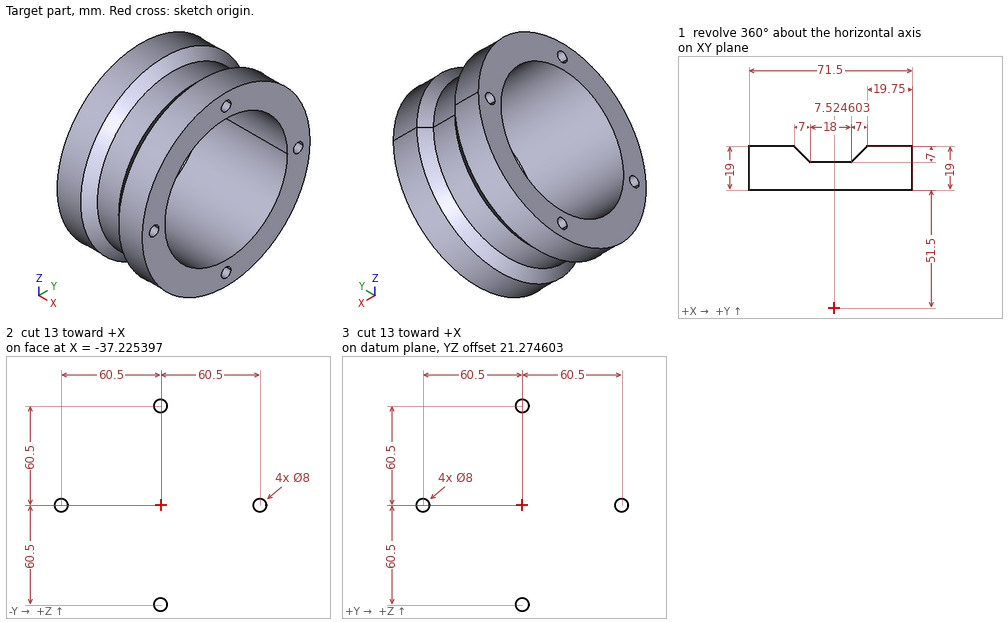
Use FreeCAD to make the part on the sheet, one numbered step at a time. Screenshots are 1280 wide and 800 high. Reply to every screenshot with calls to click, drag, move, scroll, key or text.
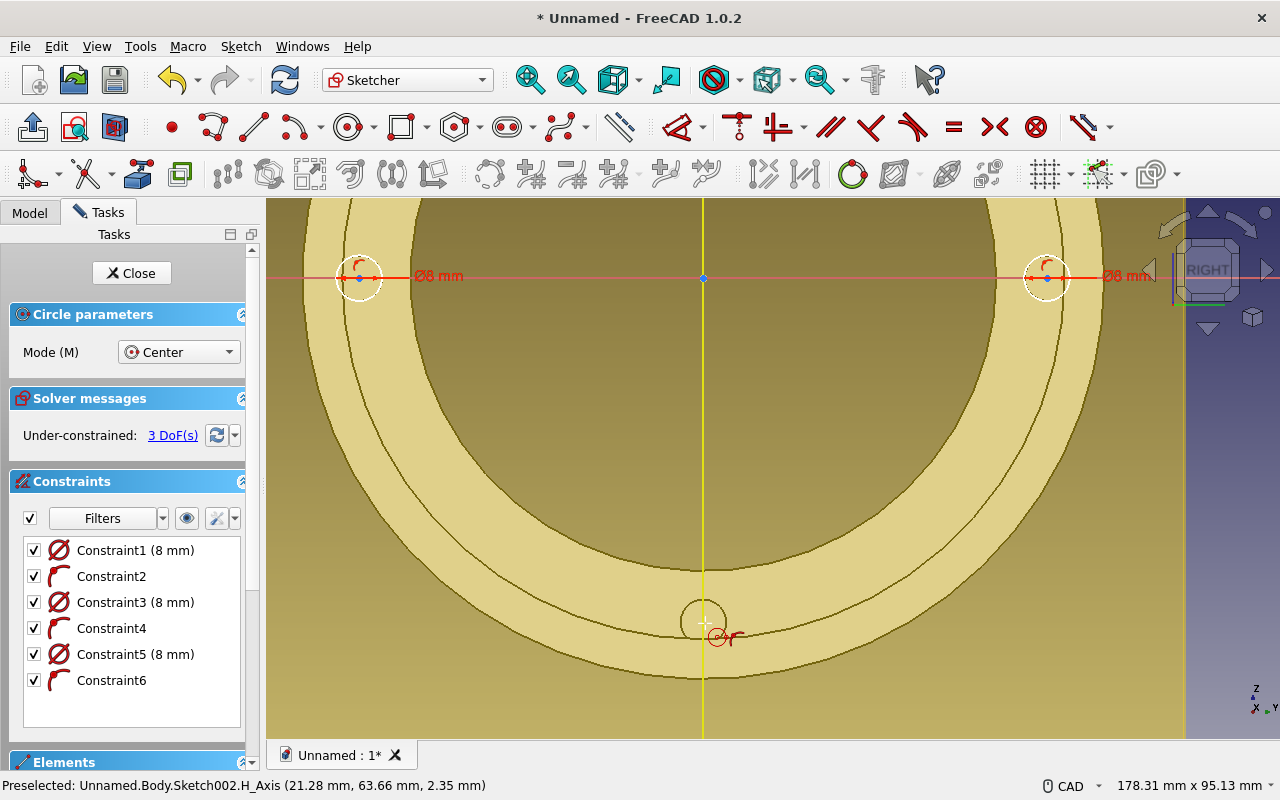
click(703, 622)
move(719, 606)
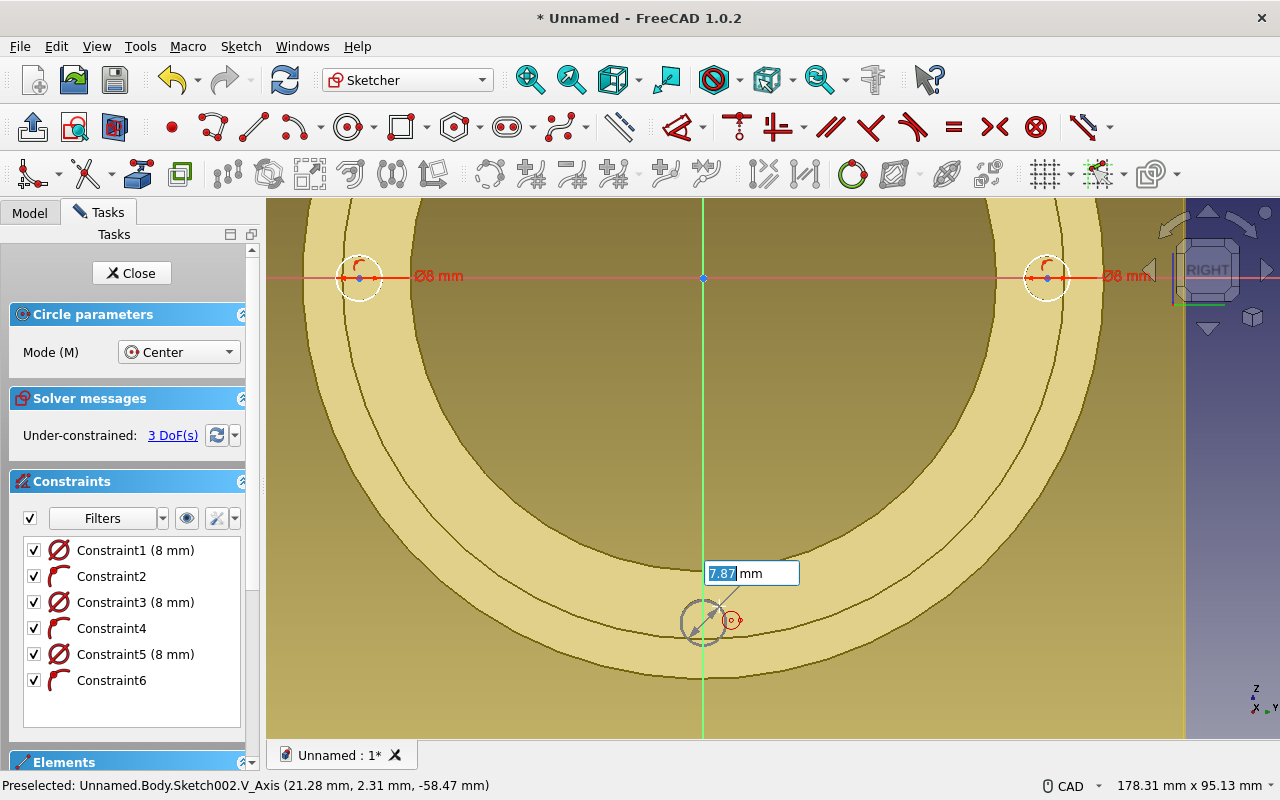
text(8)
key(Return)
key(Escape)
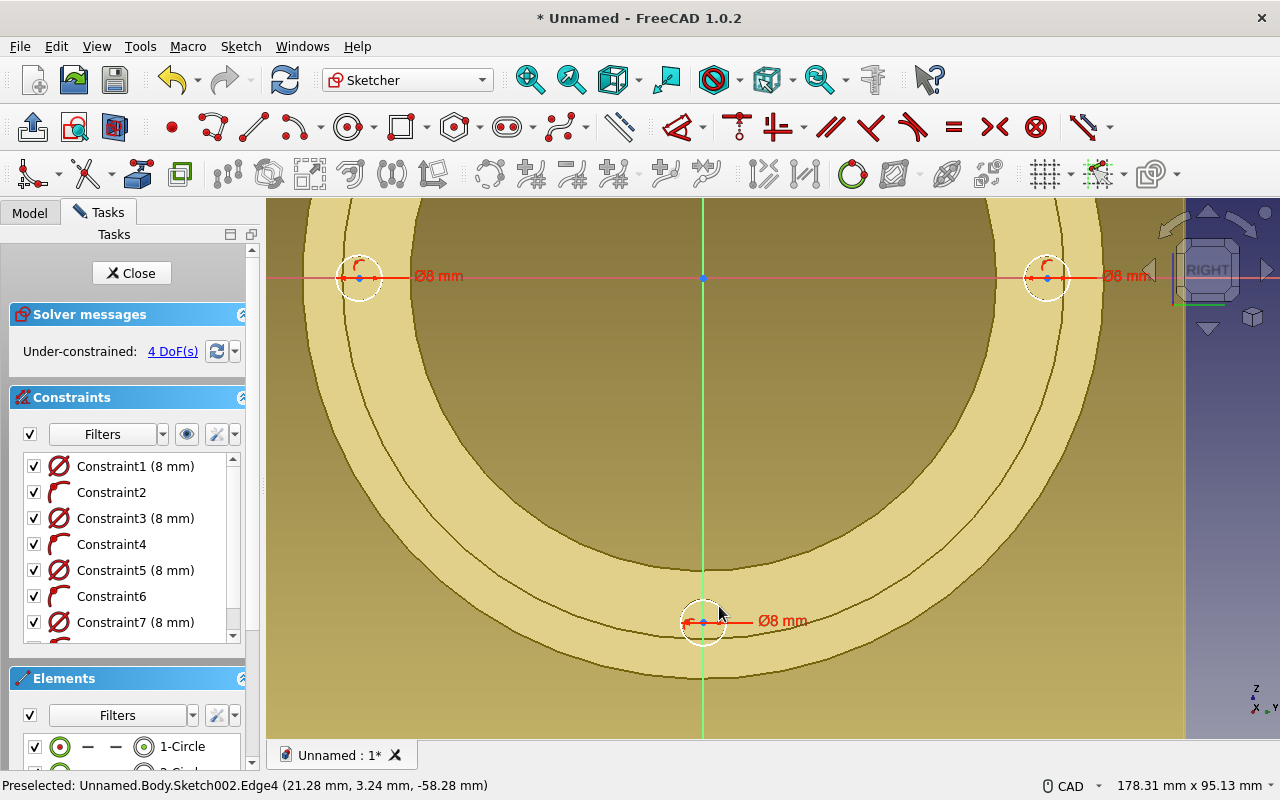
click(676, 128)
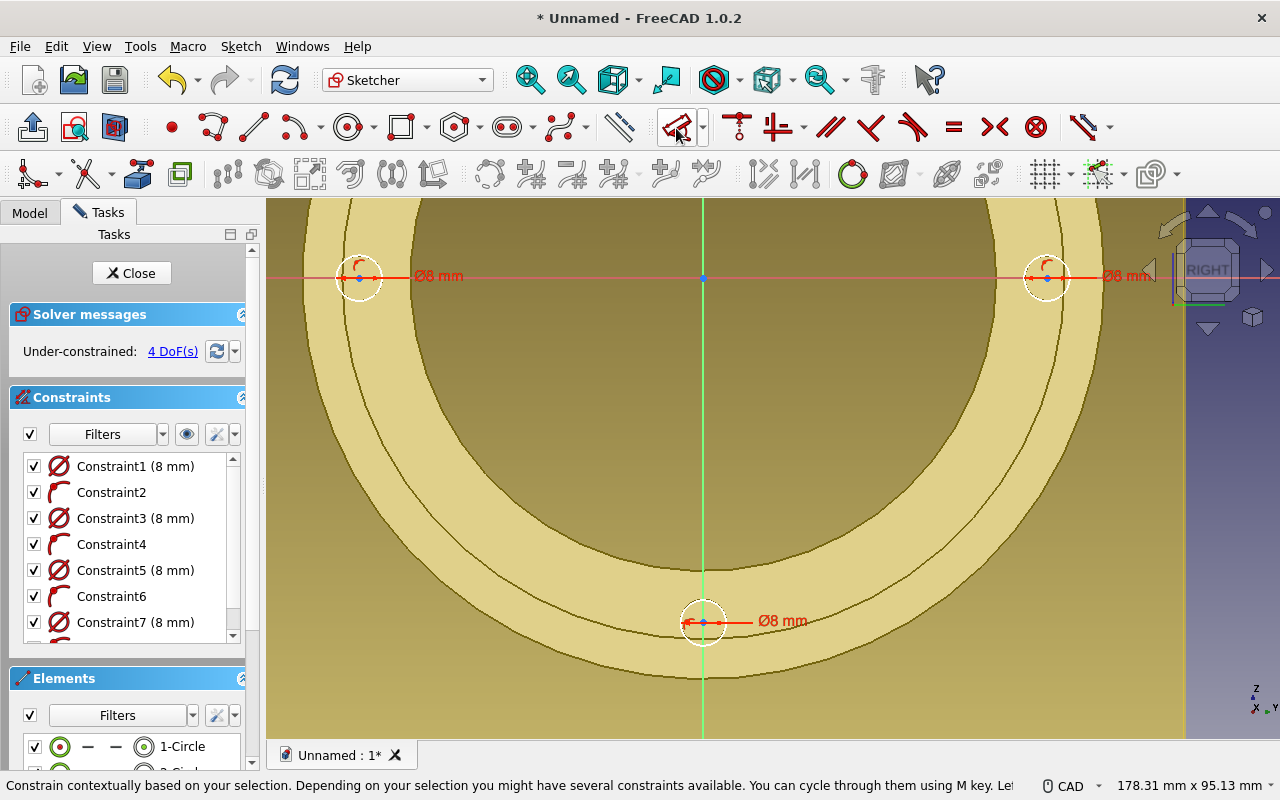
click(359, 278)
click(531, 312)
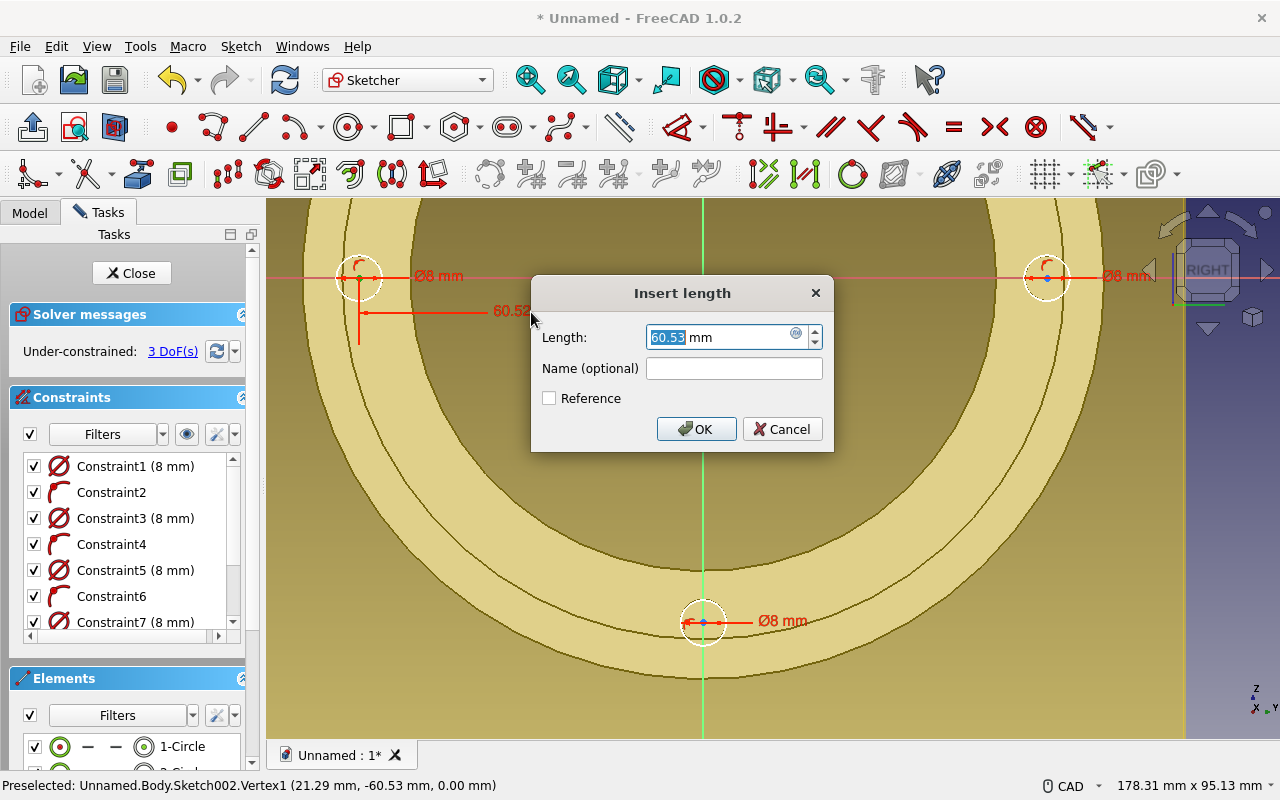
text(60.5)
key(Return)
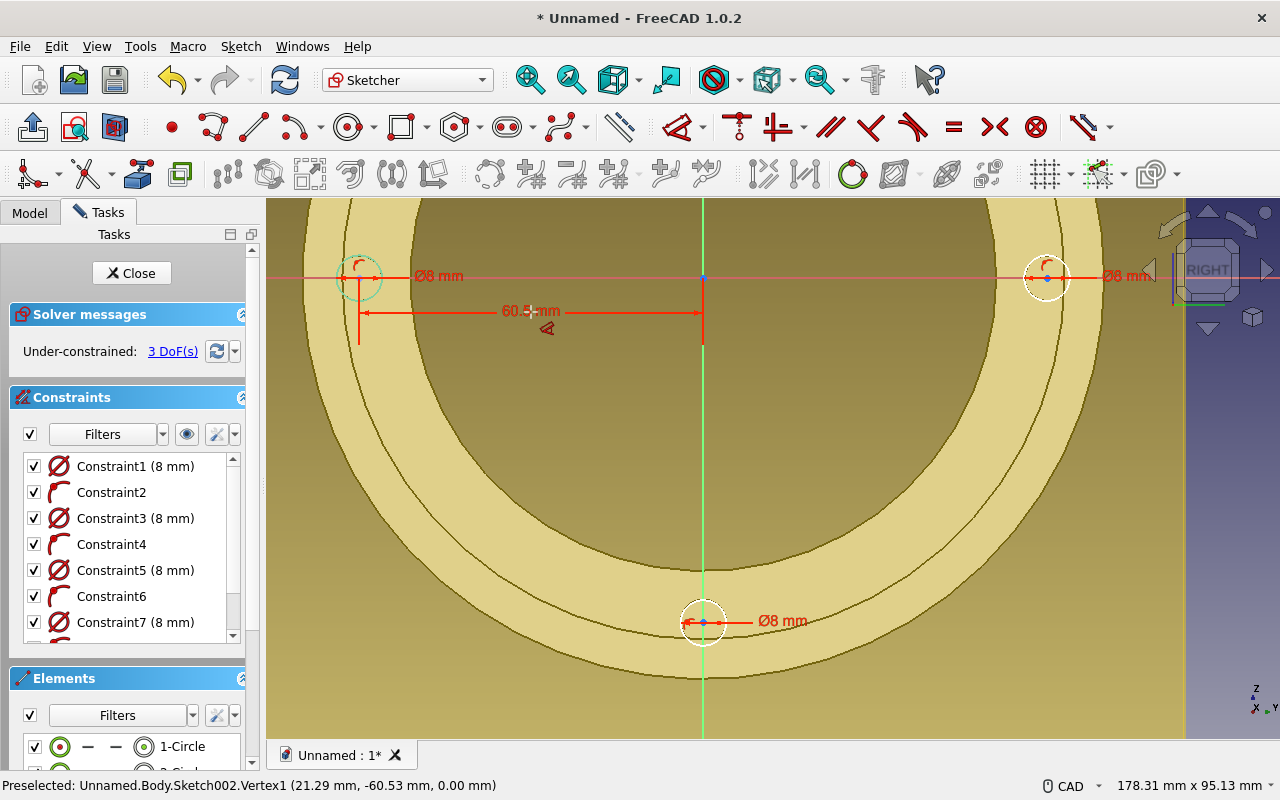
scroll(705, 624, down, 4)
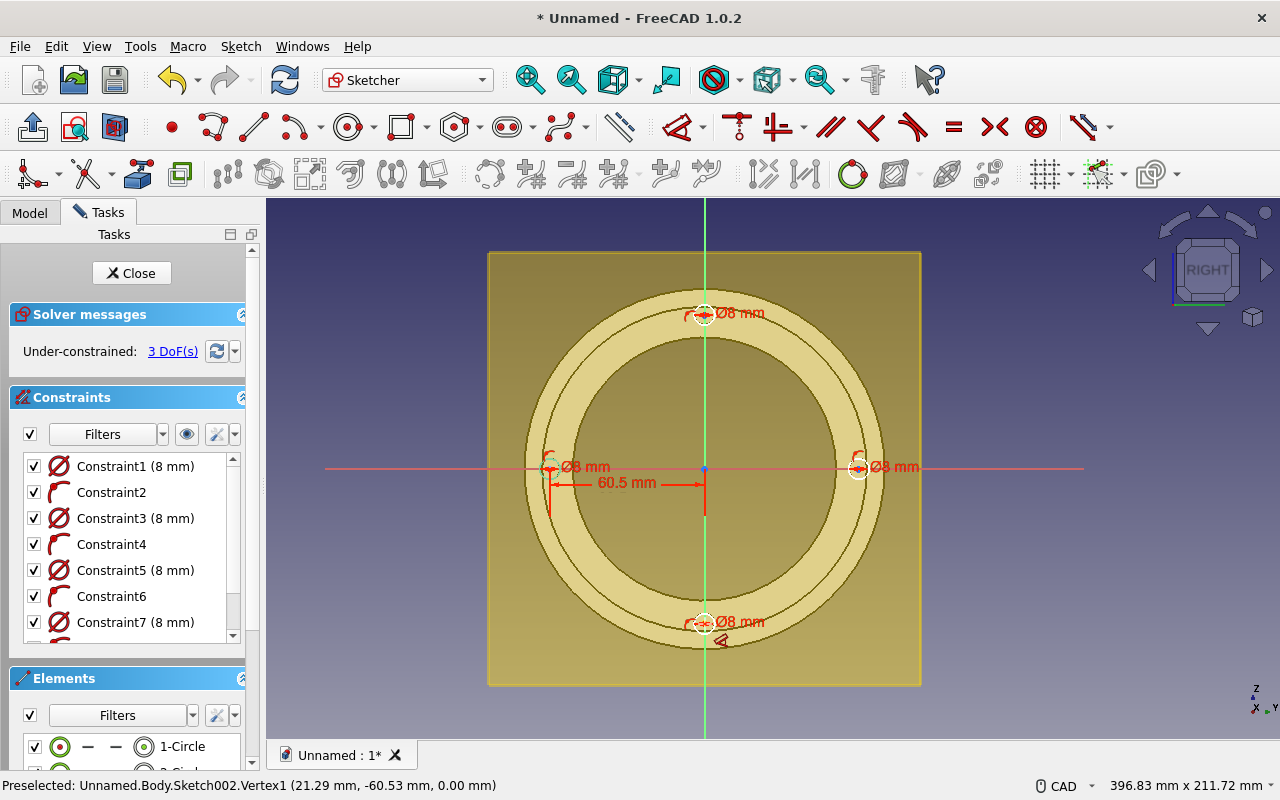
click(705, 315)
click(739, 392)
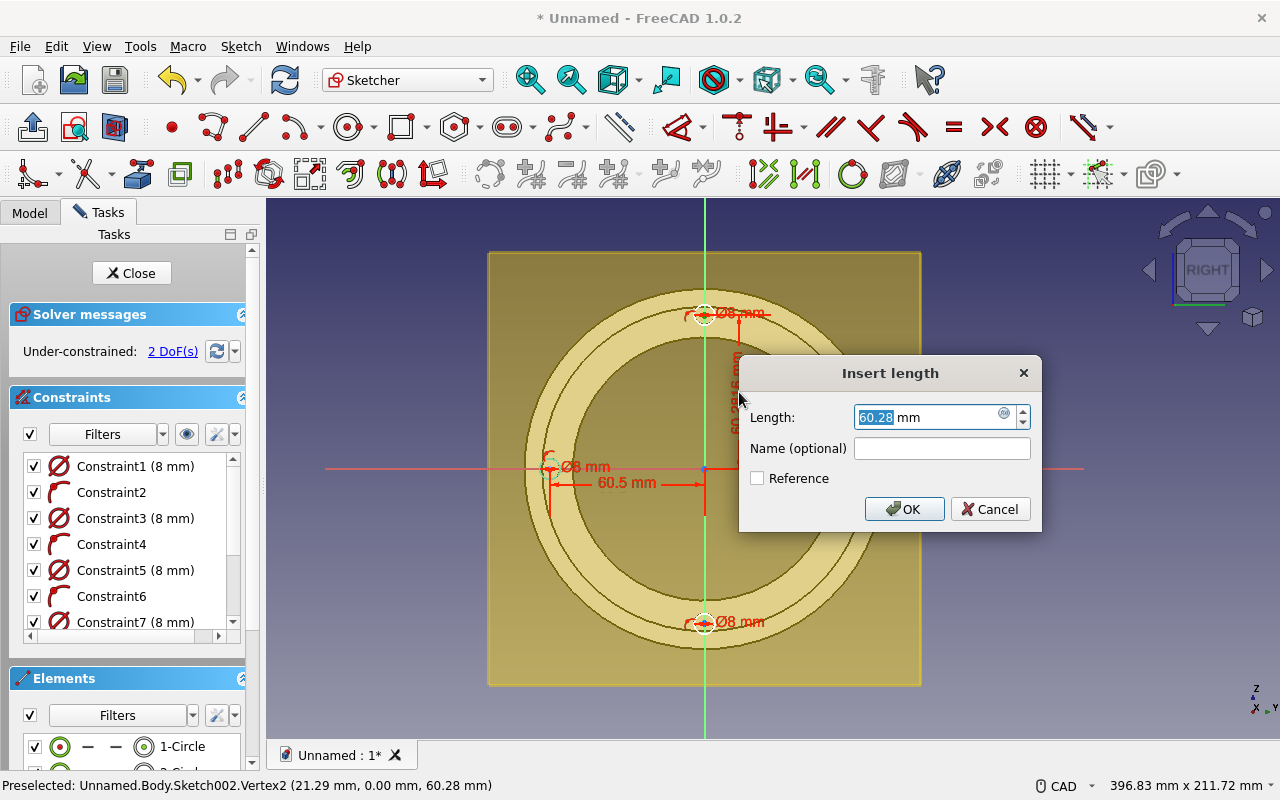
text(60.5)
key(Return)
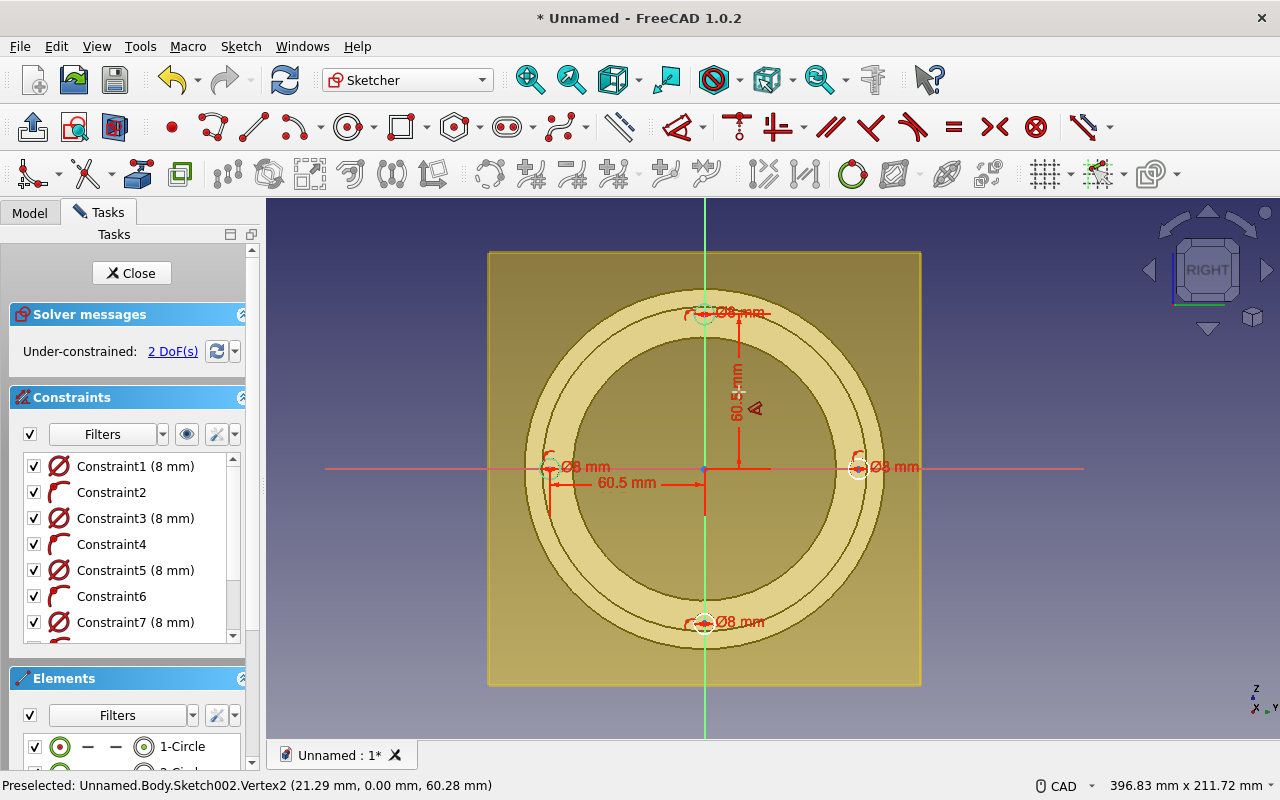
click(859, 469)
click(782, 503)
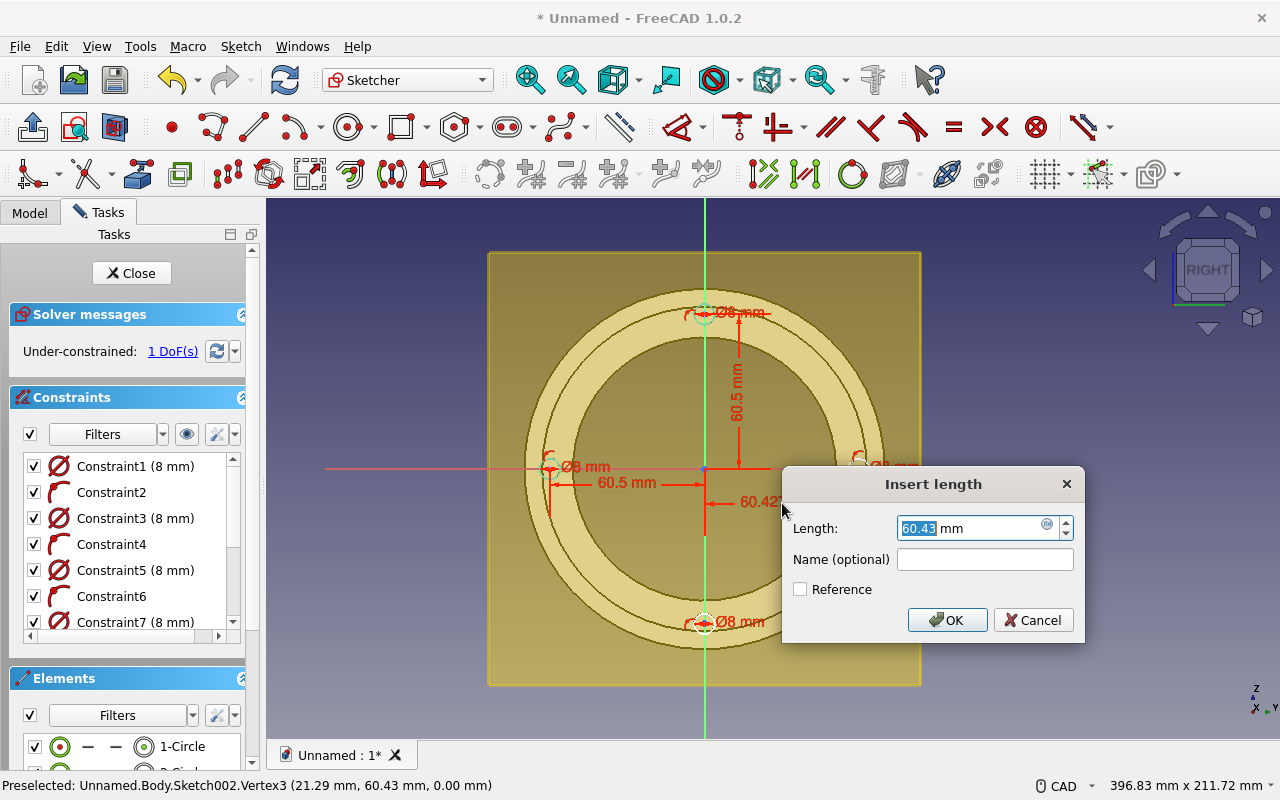
text(60.5)
key(Return)